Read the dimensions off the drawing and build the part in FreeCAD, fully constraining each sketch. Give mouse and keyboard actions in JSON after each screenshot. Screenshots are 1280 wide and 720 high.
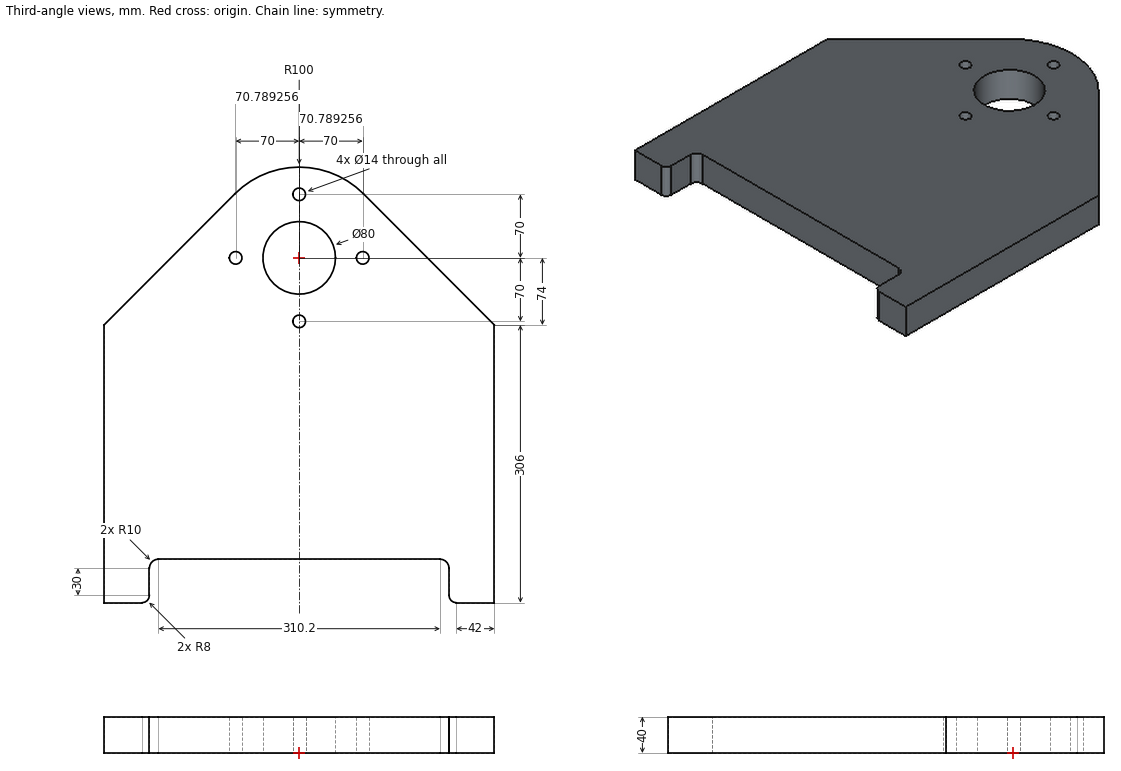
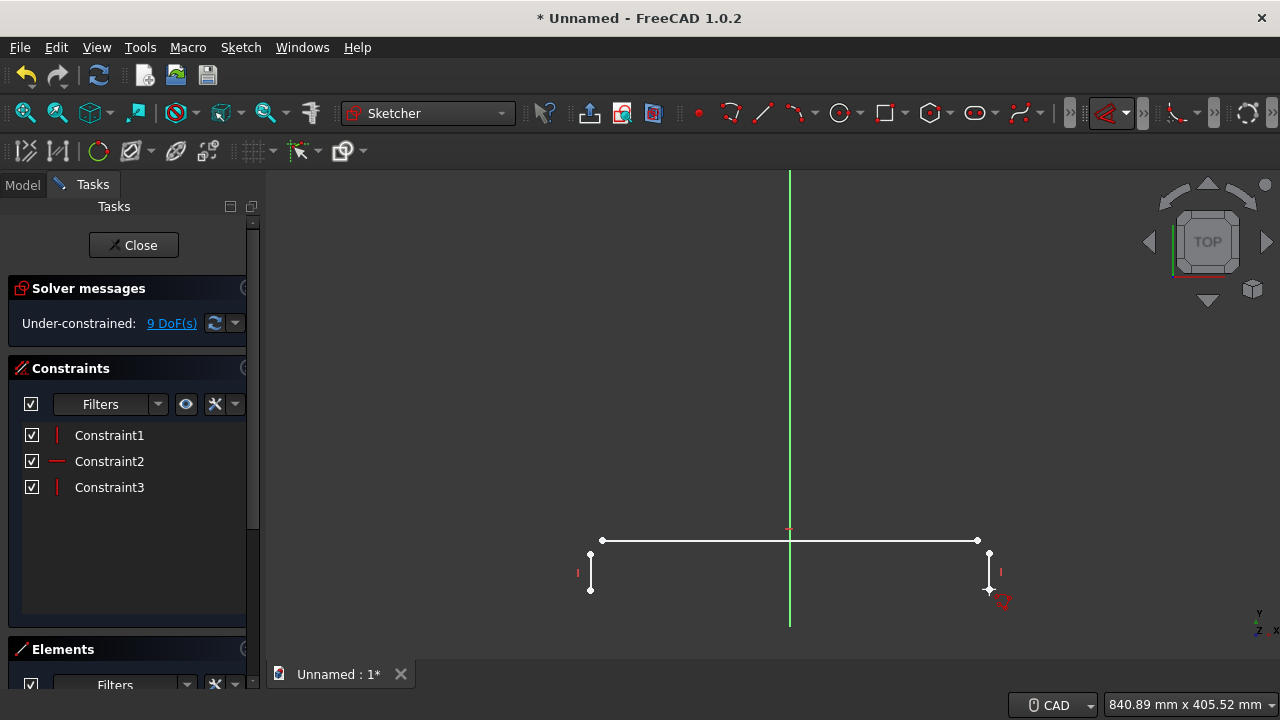
{"action": "left_click", "coordinate": [998, 598]}
{"action": "left_click", "coordinate": [1049, 598]}
{"action": "left_click", "coordinate": [1049, 229]}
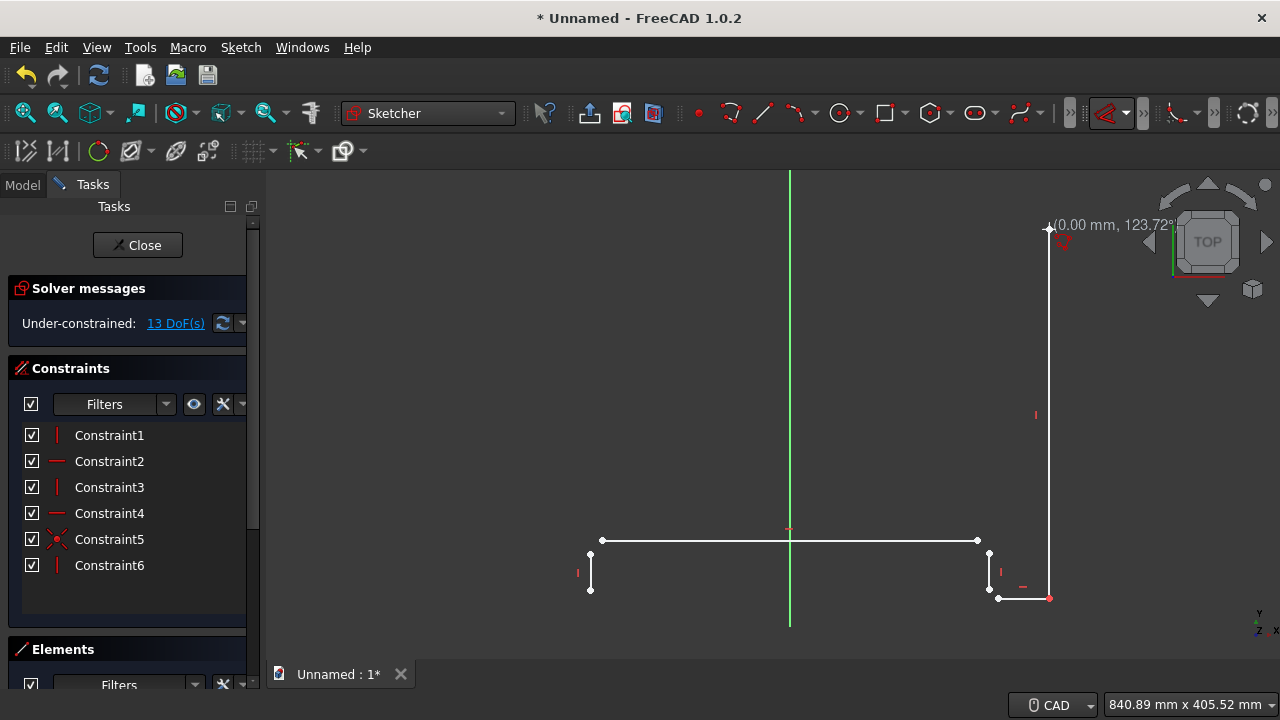
{"action": "scroll", "coordinate": [601, 543], "scroll_direction": "down", "scroll_amount": 3}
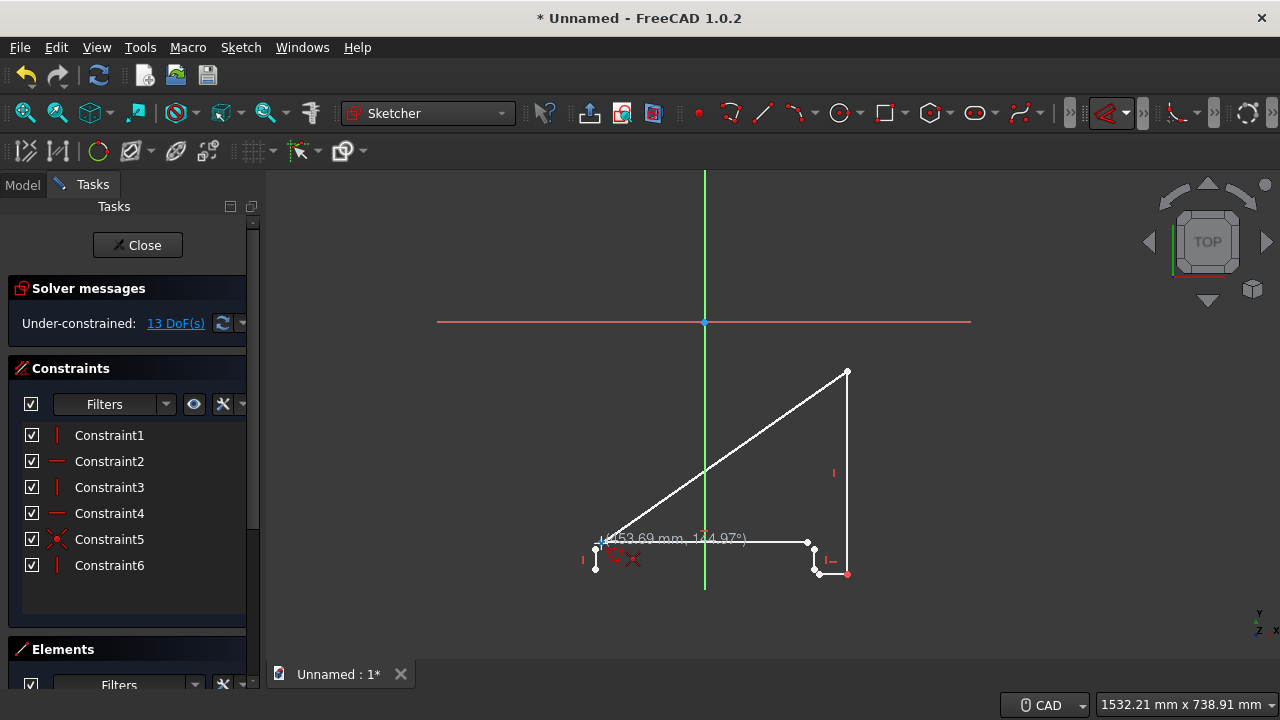
{"action": "left_click", "coordinate": [751, 275]}
{"action": "right_click", "coordinate": [751, 275]}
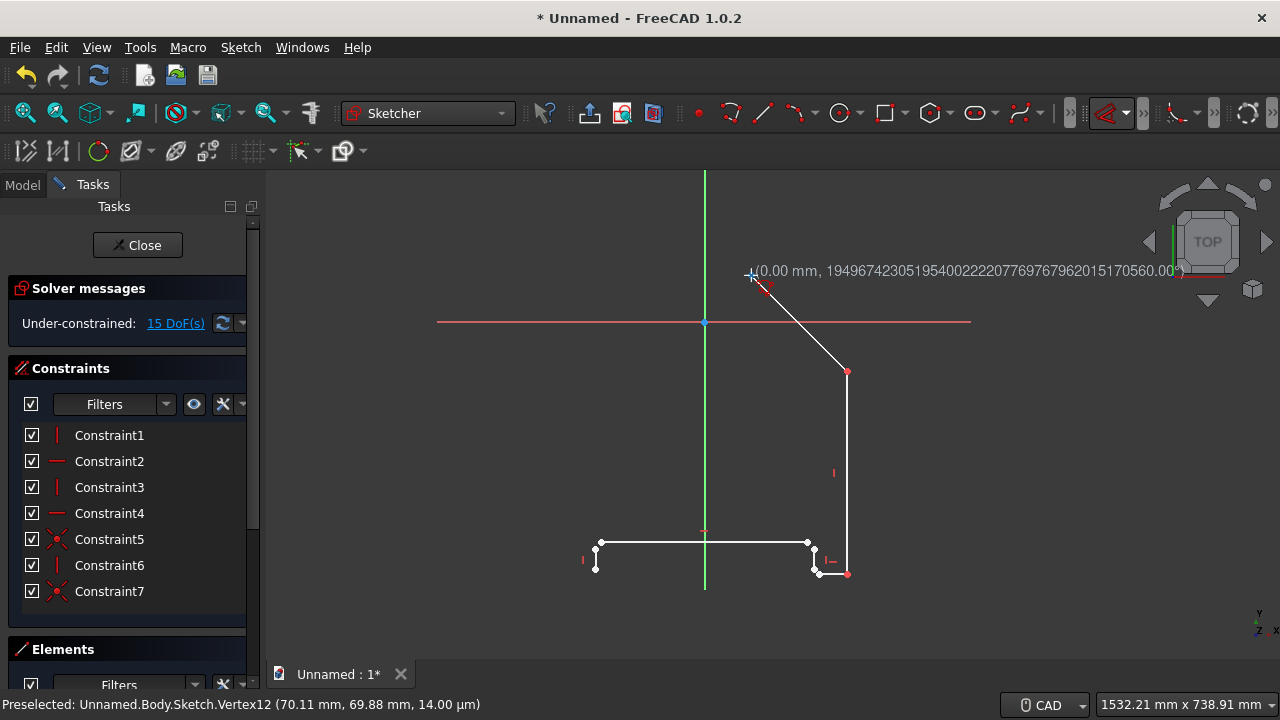
{"action": "left_click", "coordinate": [658, 275]}
{"action": "left_click", "coordinate": [562, 371]}
{"action": "left_click", "coordinate": [562, 574]}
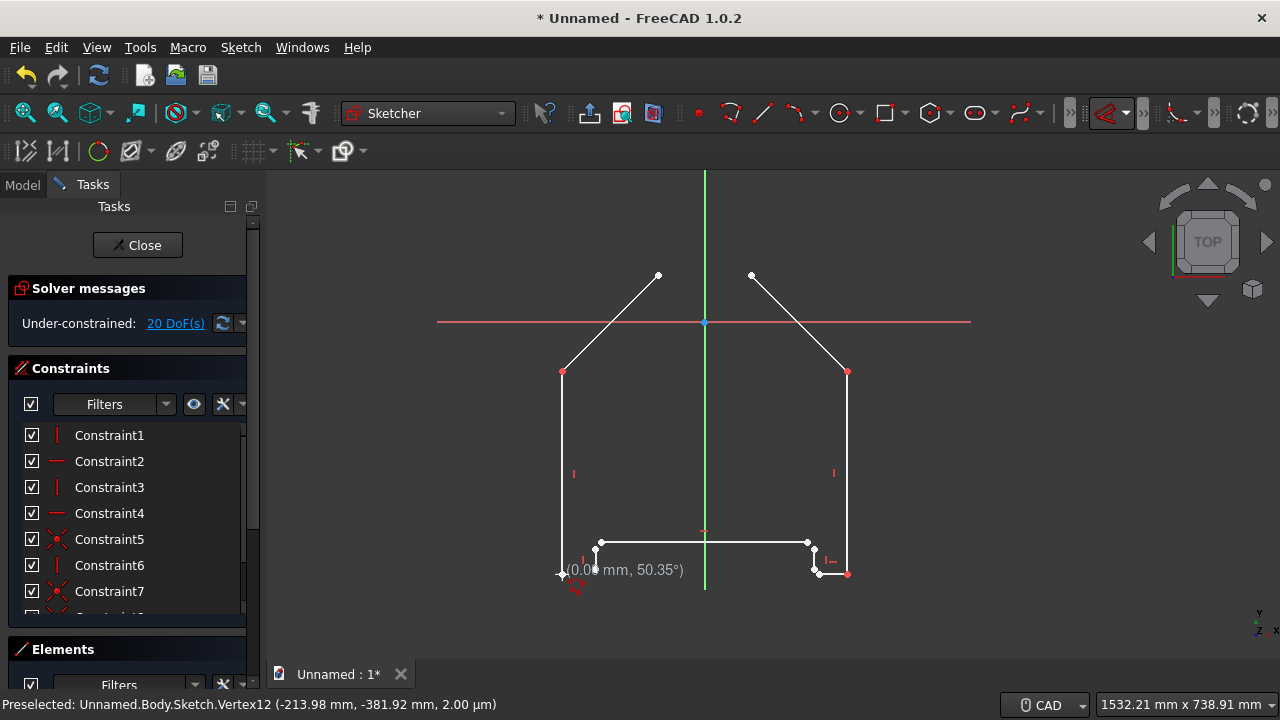
{"action": "scroll", "coordinate": [590, 574], "scroll_direction": "up", "scroll_amount": 4}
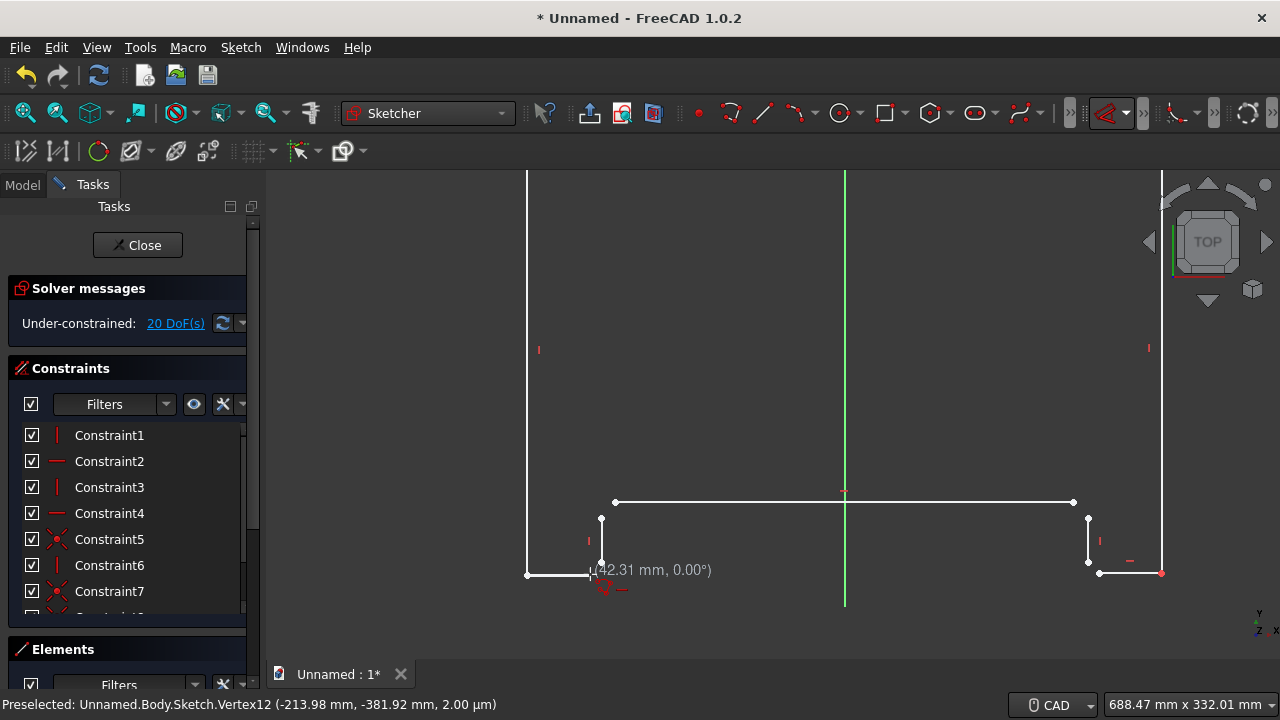
{"action": "left_click", "coordinate": [590, 573]}
{"action": "right_click", "coordinate": [590, 573]}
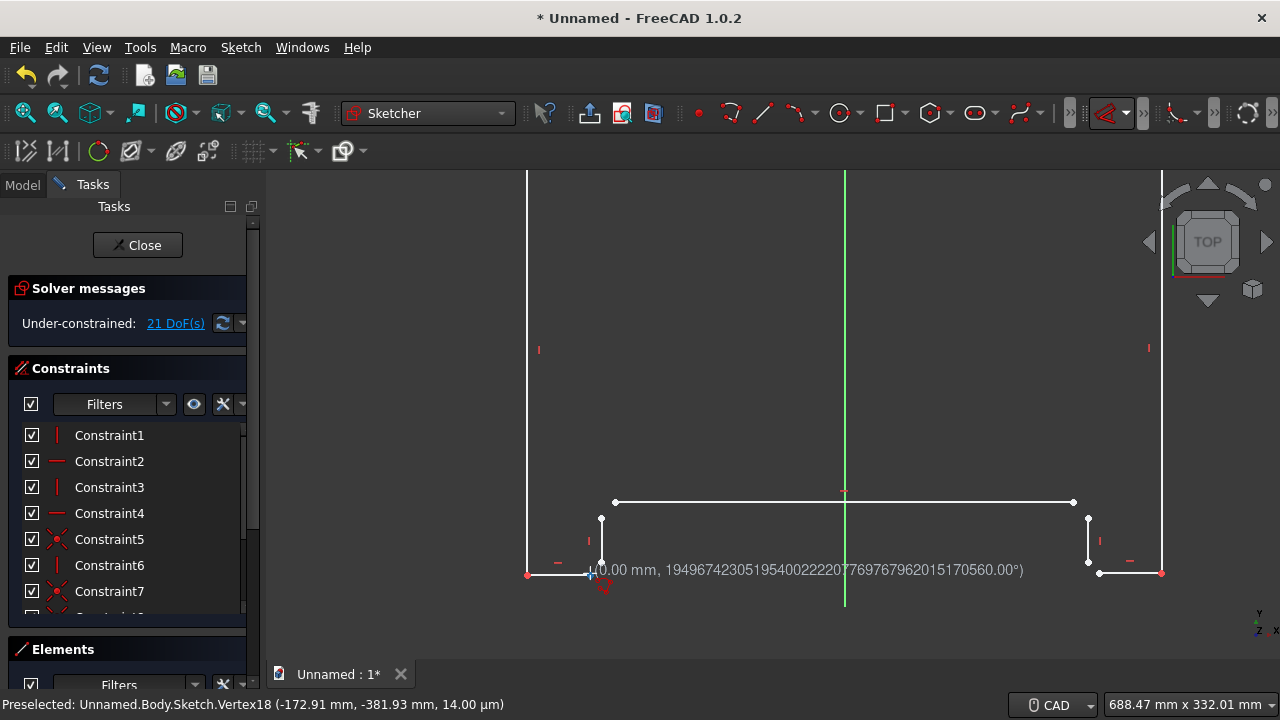
{"action": "key", "text": "g 3 a"}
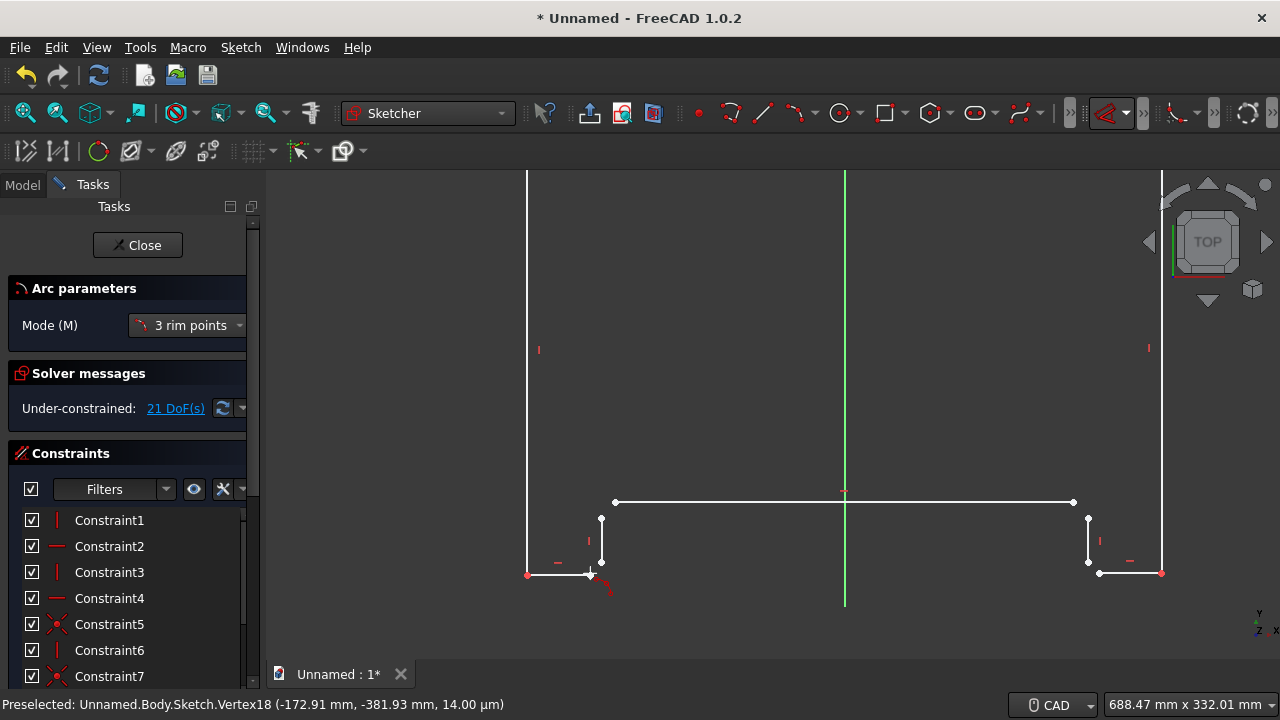
{"action": "left_click", "coordinate": [602, 518]}
{"action": "left_click", "coordinate": [616, 502]}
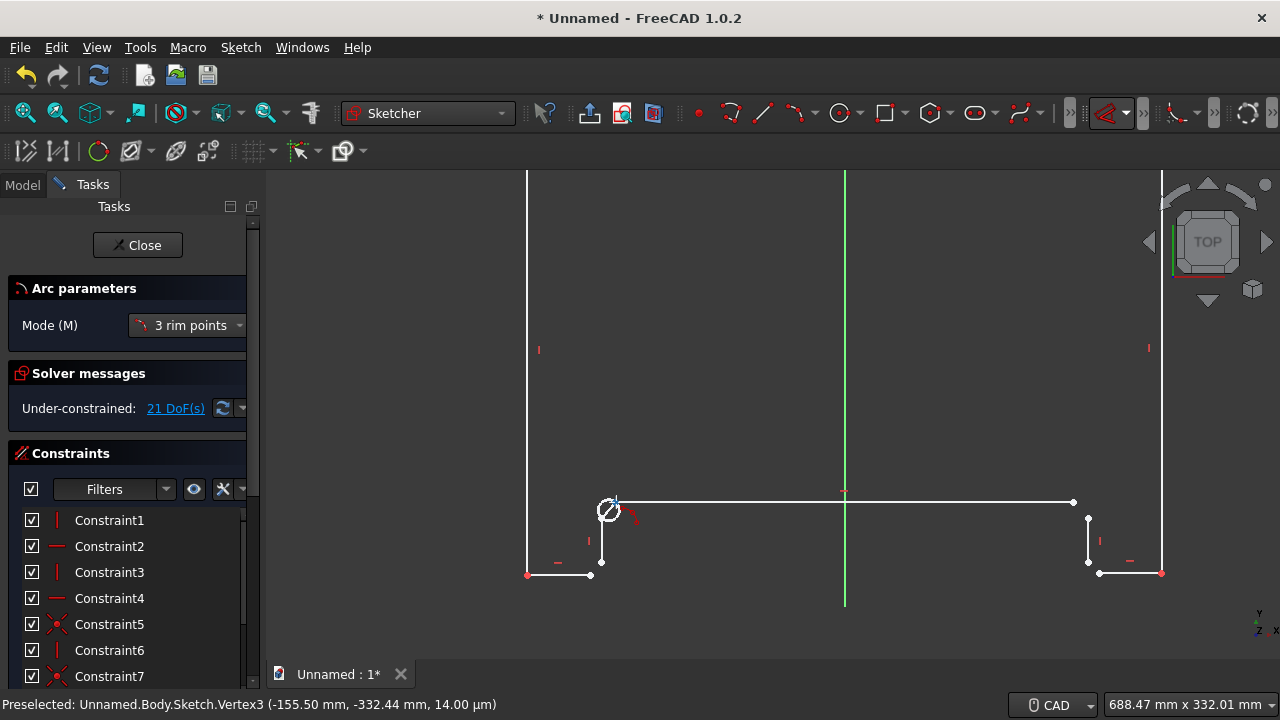
{"action": "scroll", "coordinate": [606, 506], "scroll_direction": "up", "scroll_amount": 7}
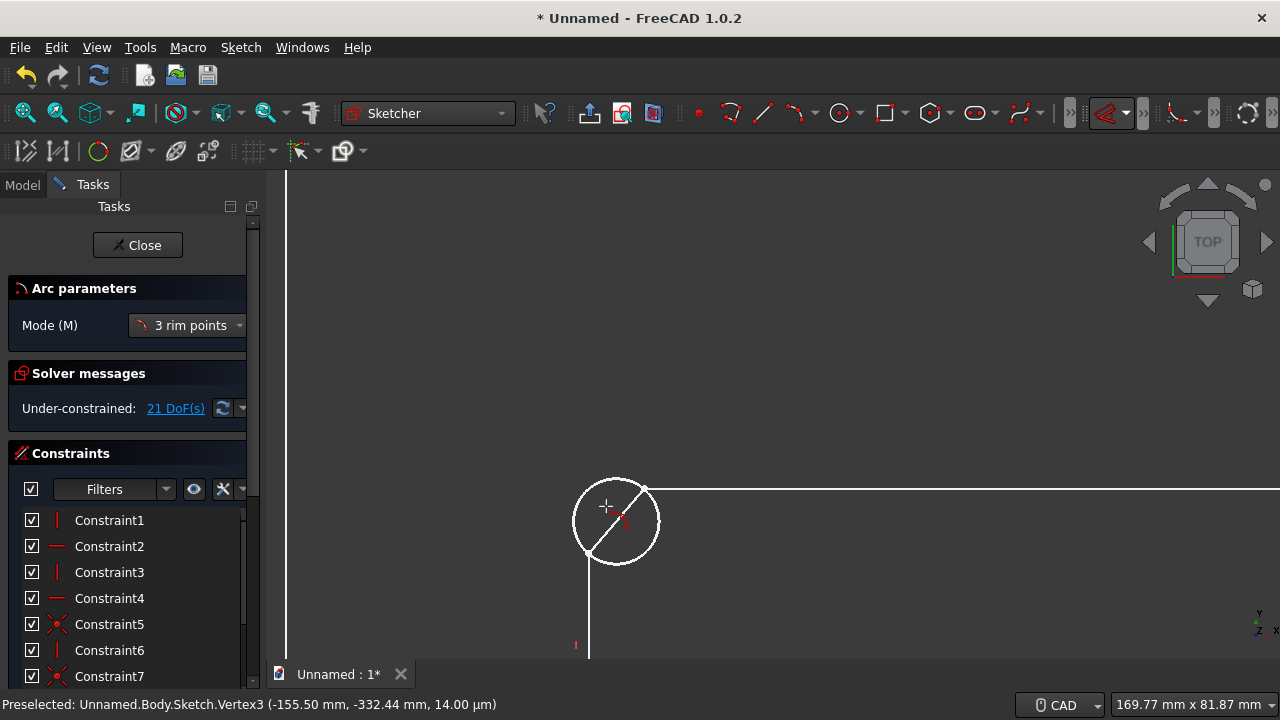
{"action": "left_click", "coordinate": [604, 504]}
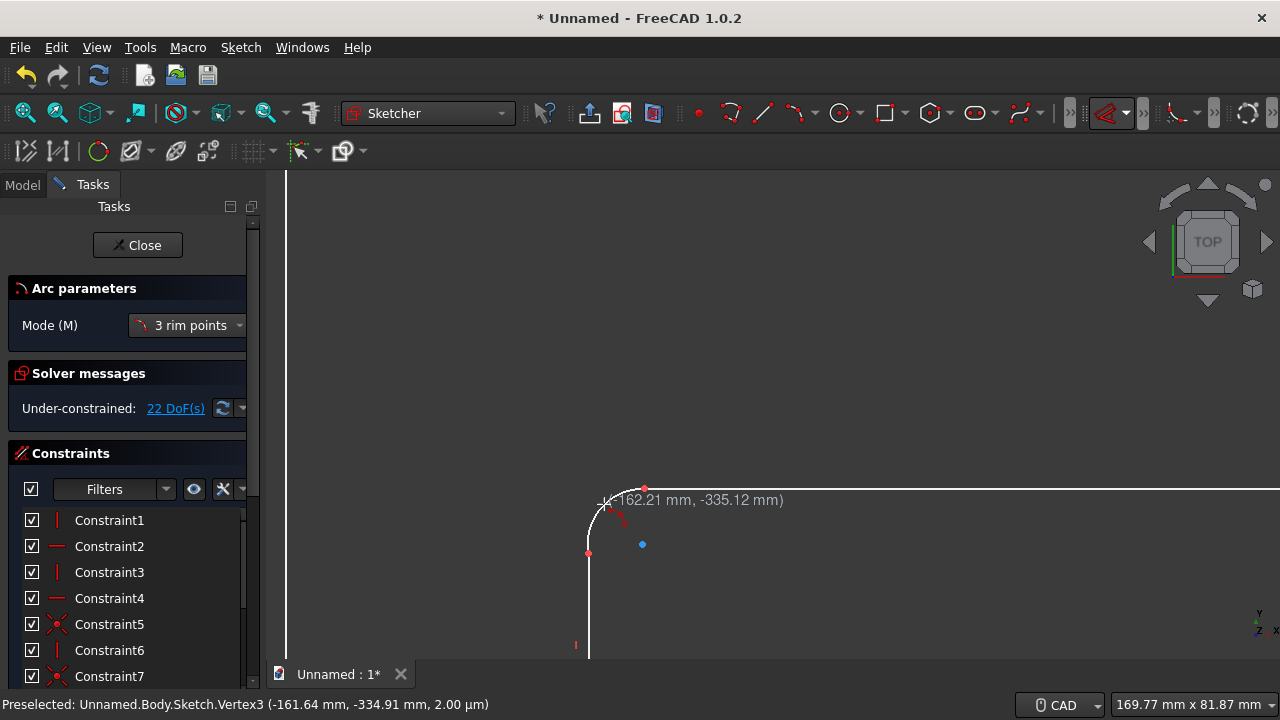
{"action": "scroll", "coordinate": [596, 548], "scroll_direction": "down", "scroll_amount": 11}